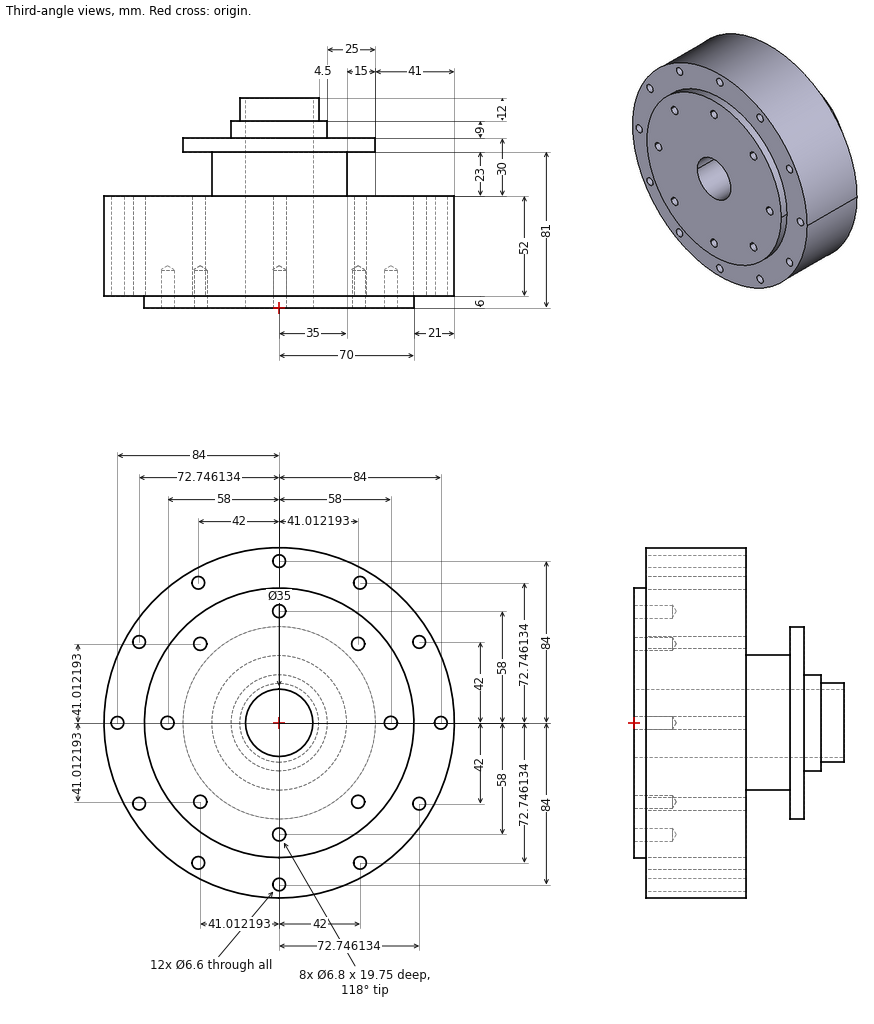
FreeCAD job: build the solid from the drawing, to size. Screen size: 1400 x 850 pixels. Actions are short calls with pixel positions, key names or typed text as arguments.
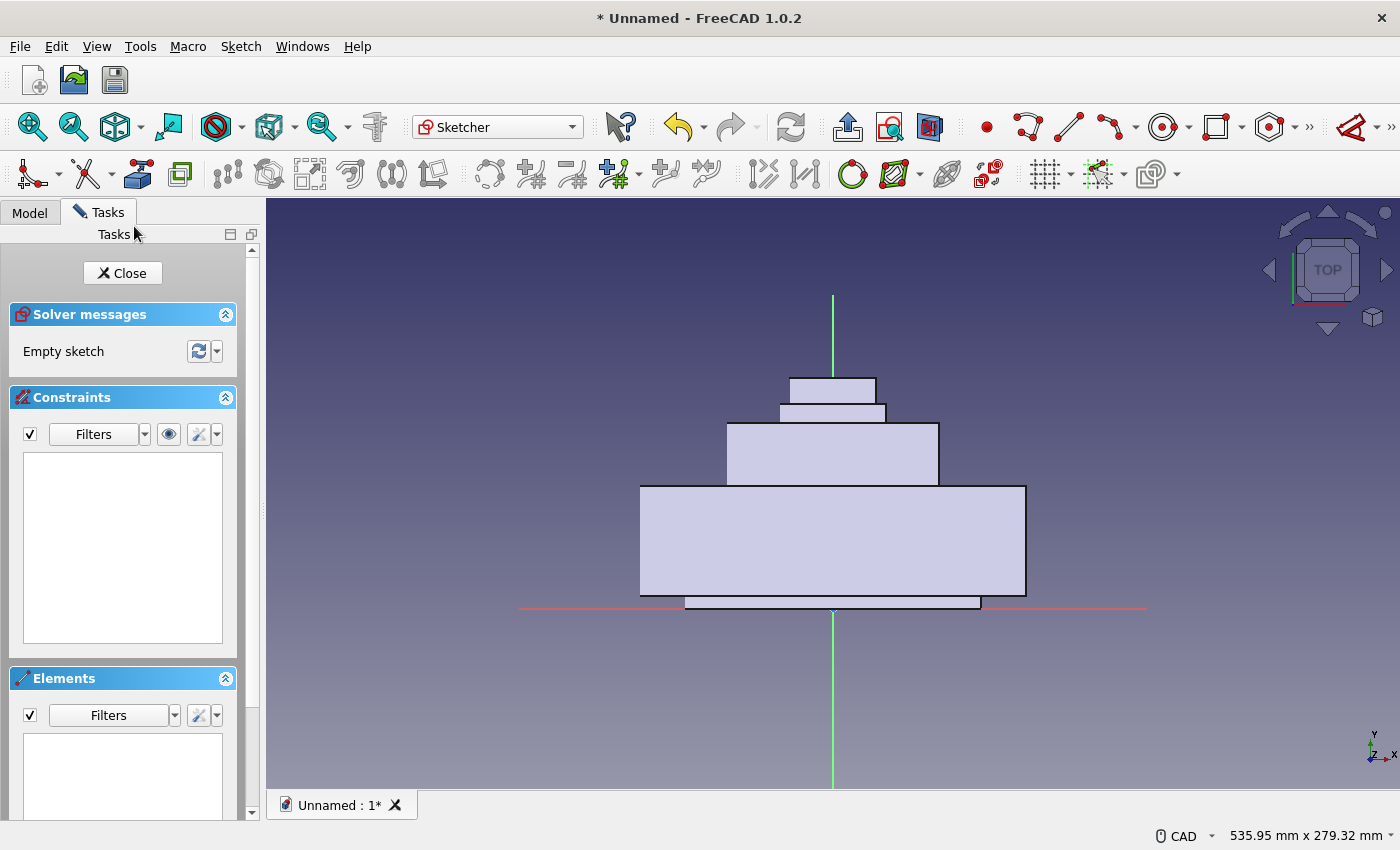
key(q)
key(s)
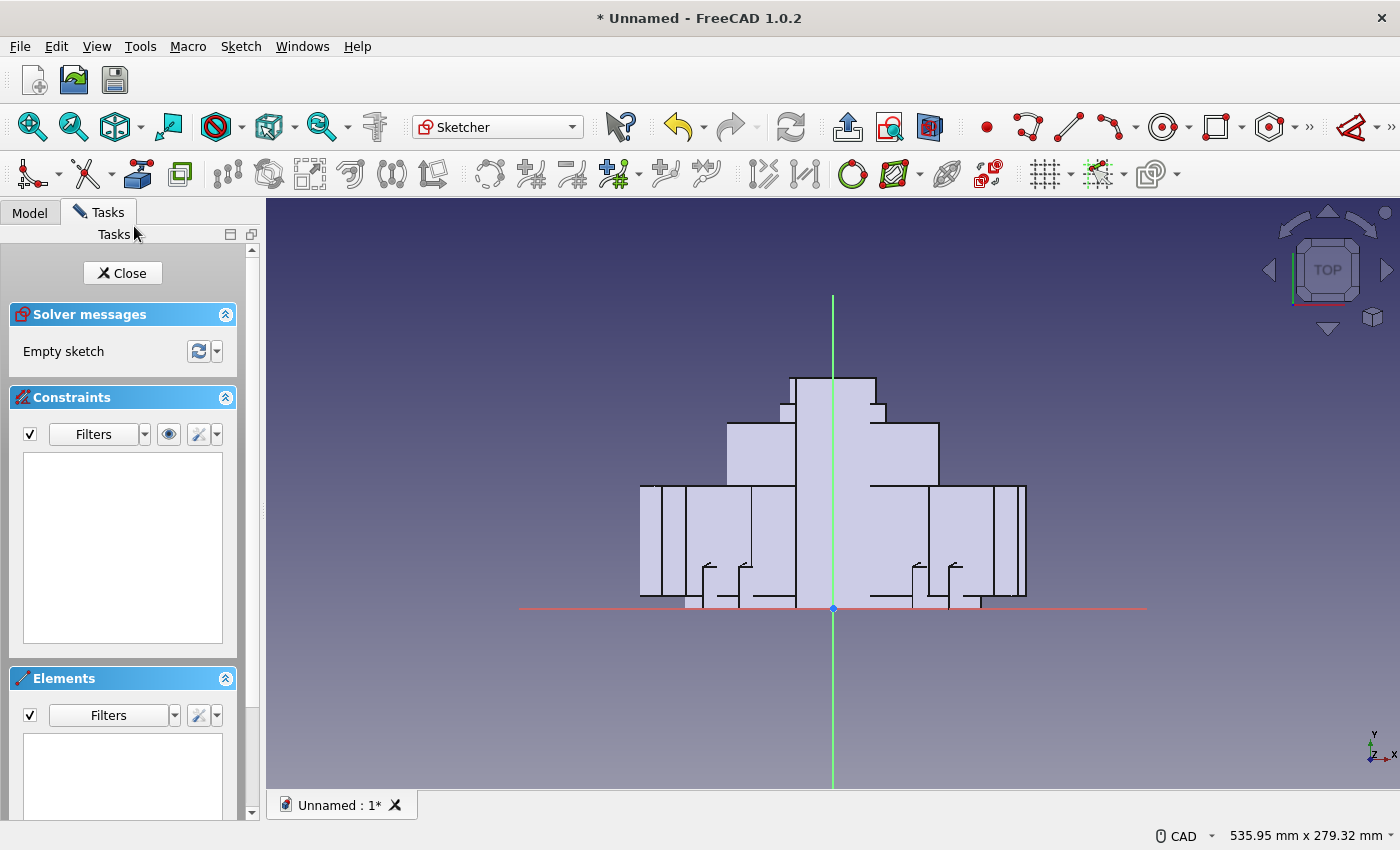
scroll(948, 457, up, 10)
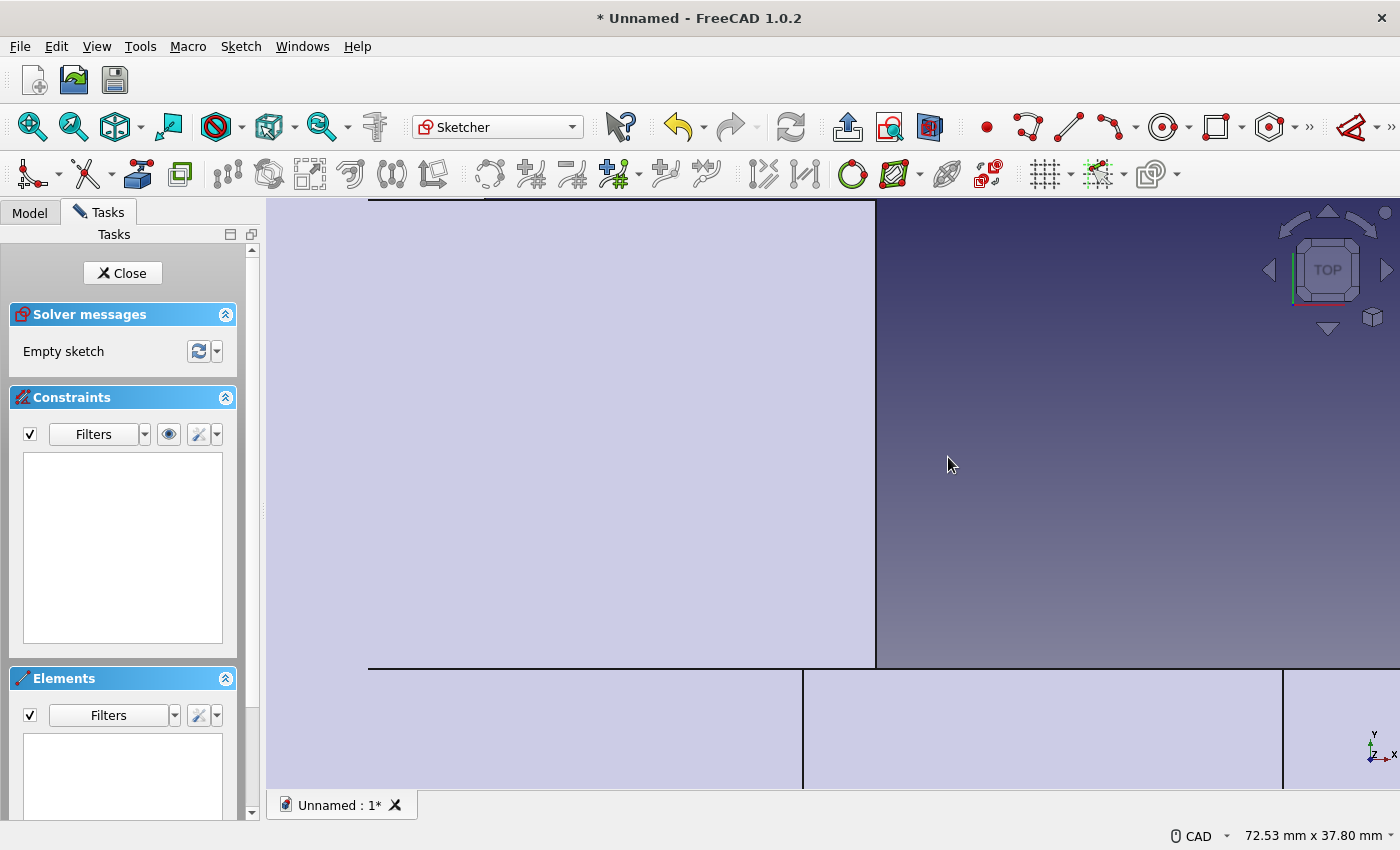
click(1216, 128)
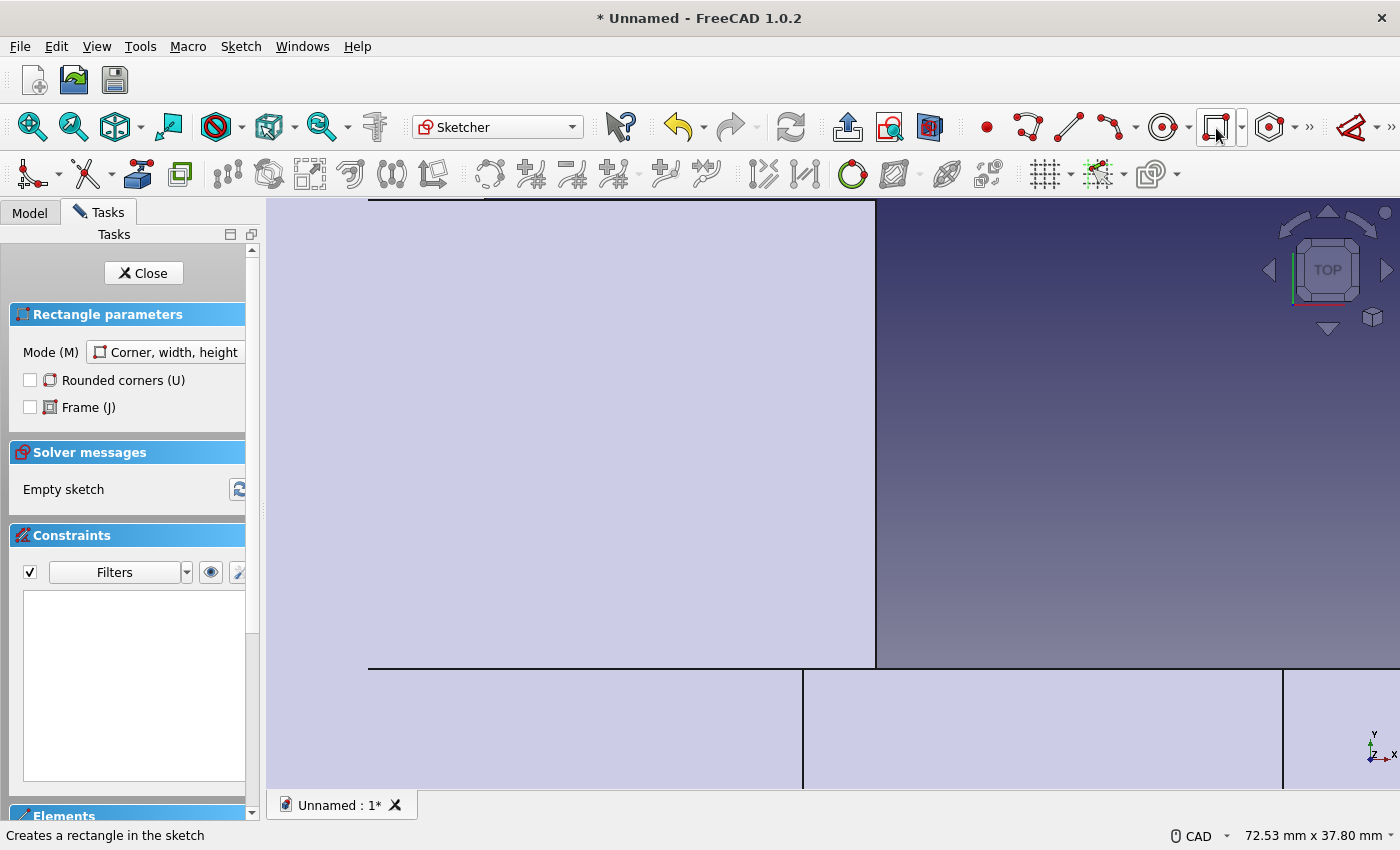
click(642, 310)
click(876, 669)
key(Escape)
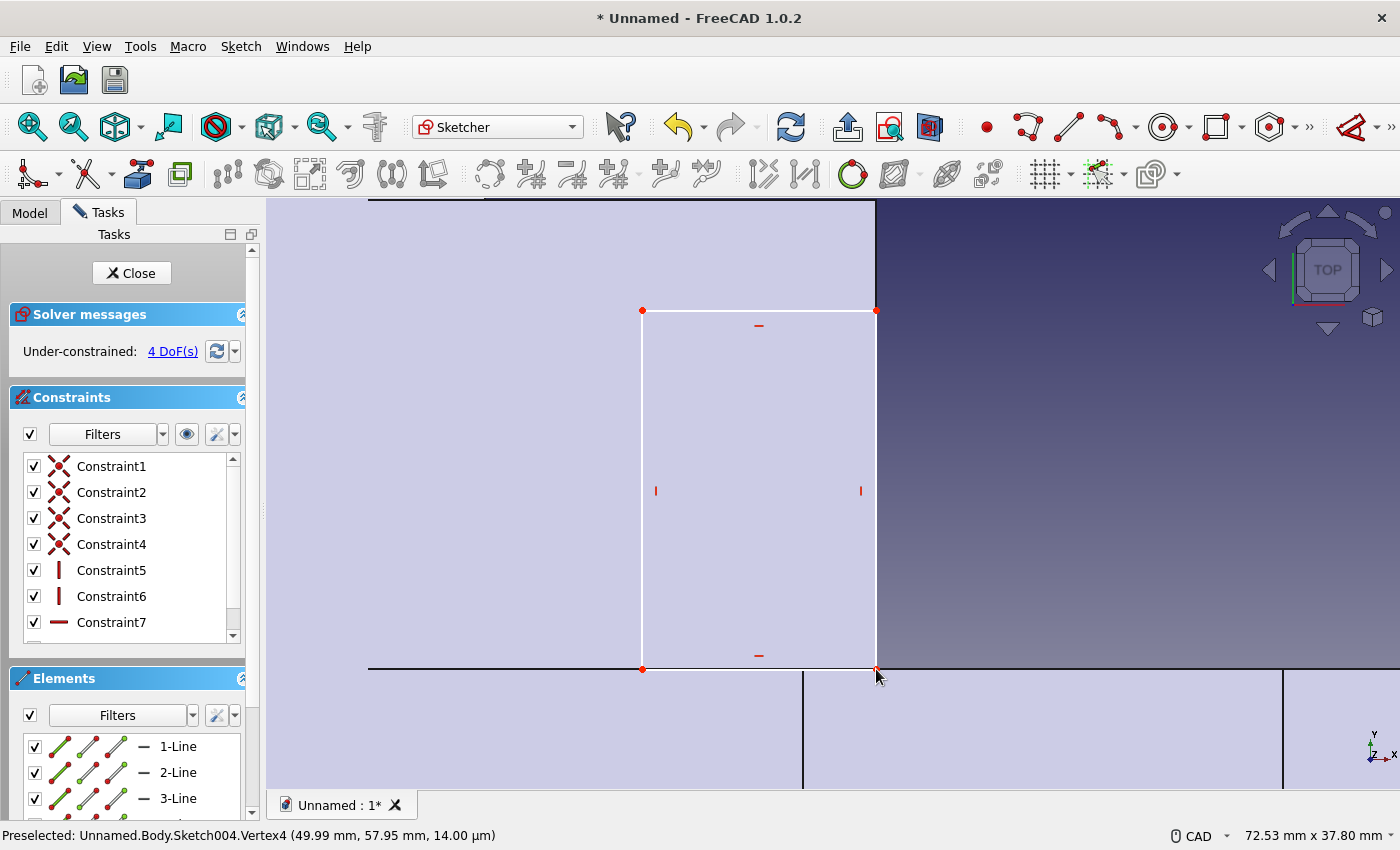
key(d)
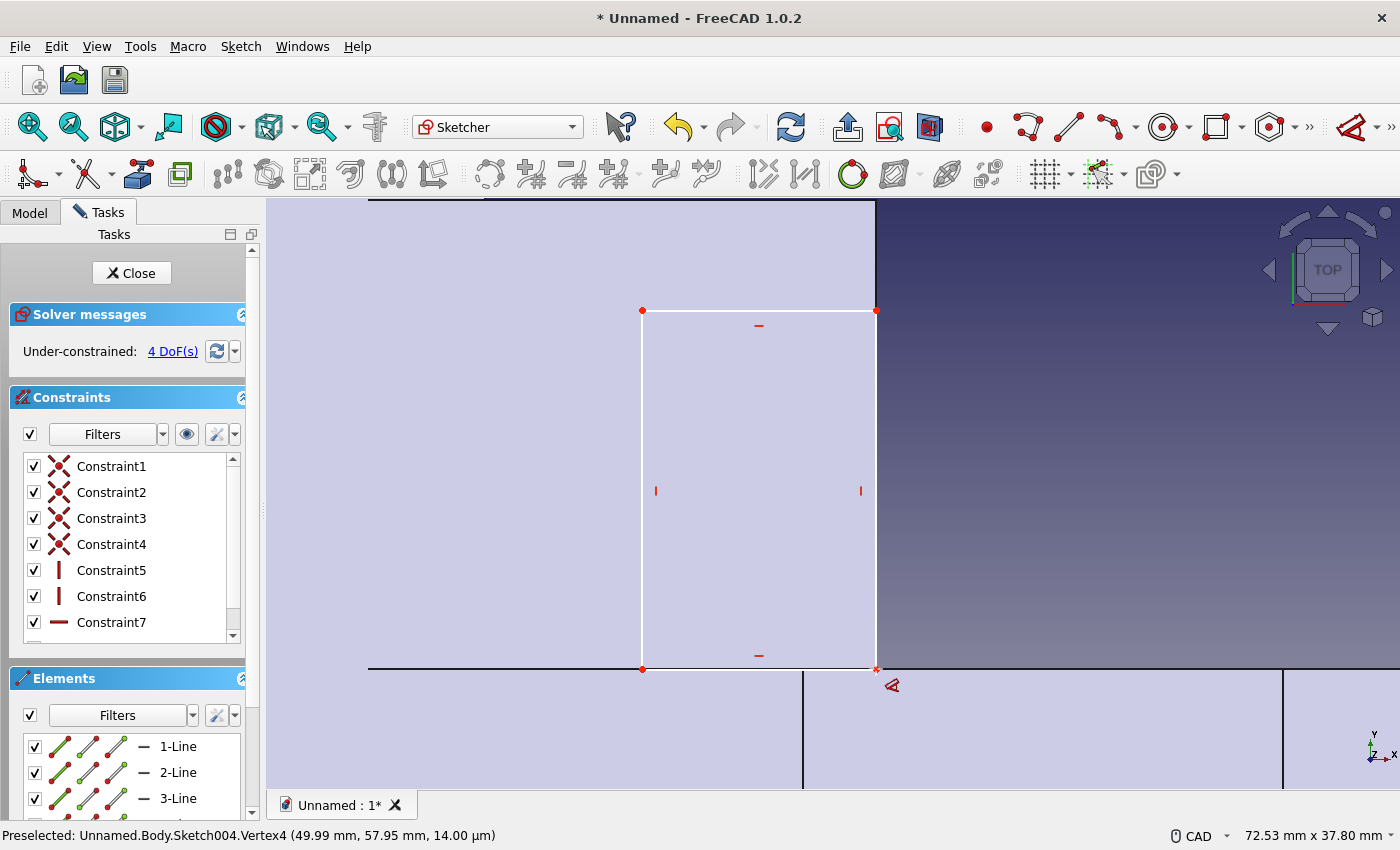
click(642, 419)
click(608, 490)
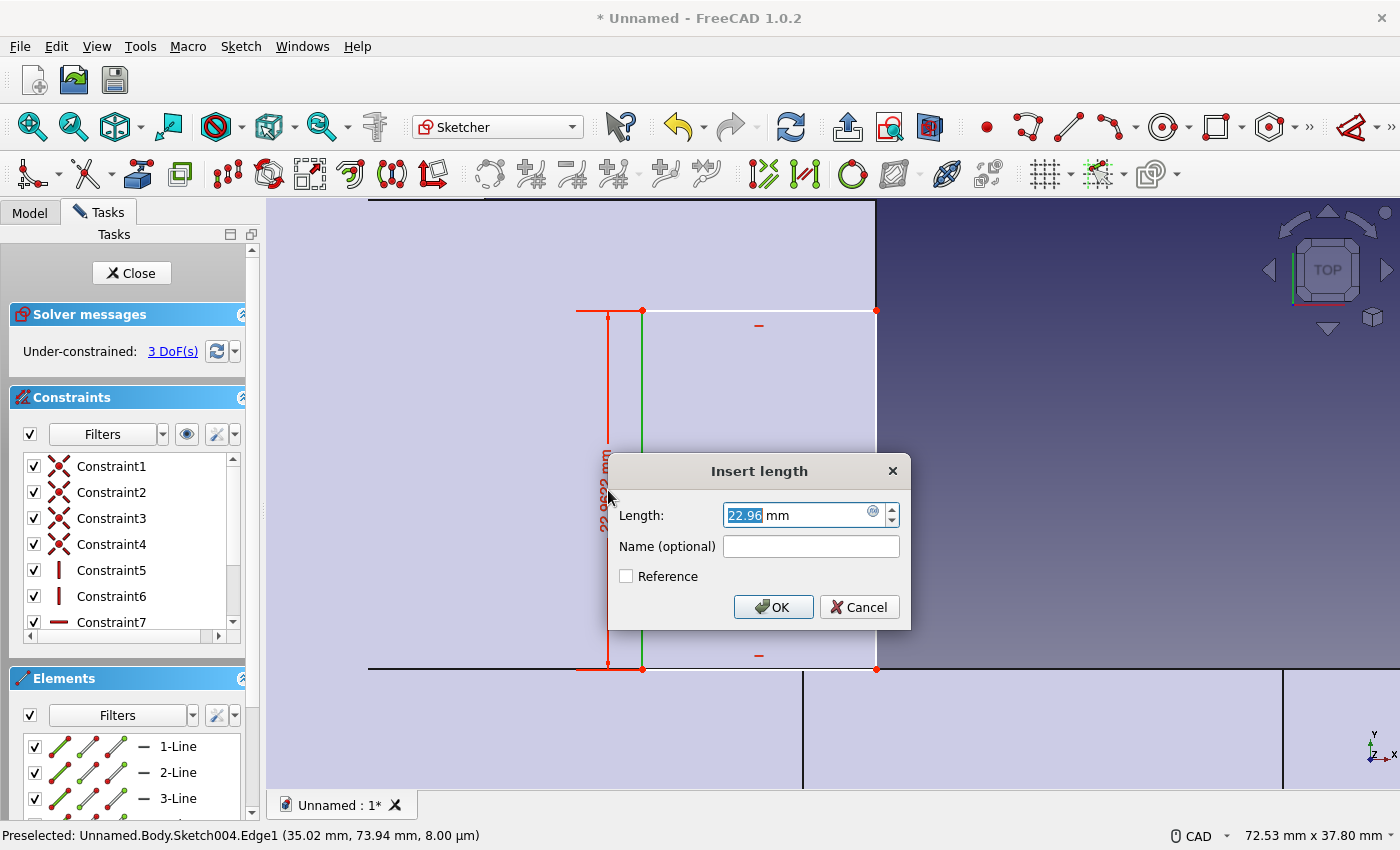
text(23)
key(Return)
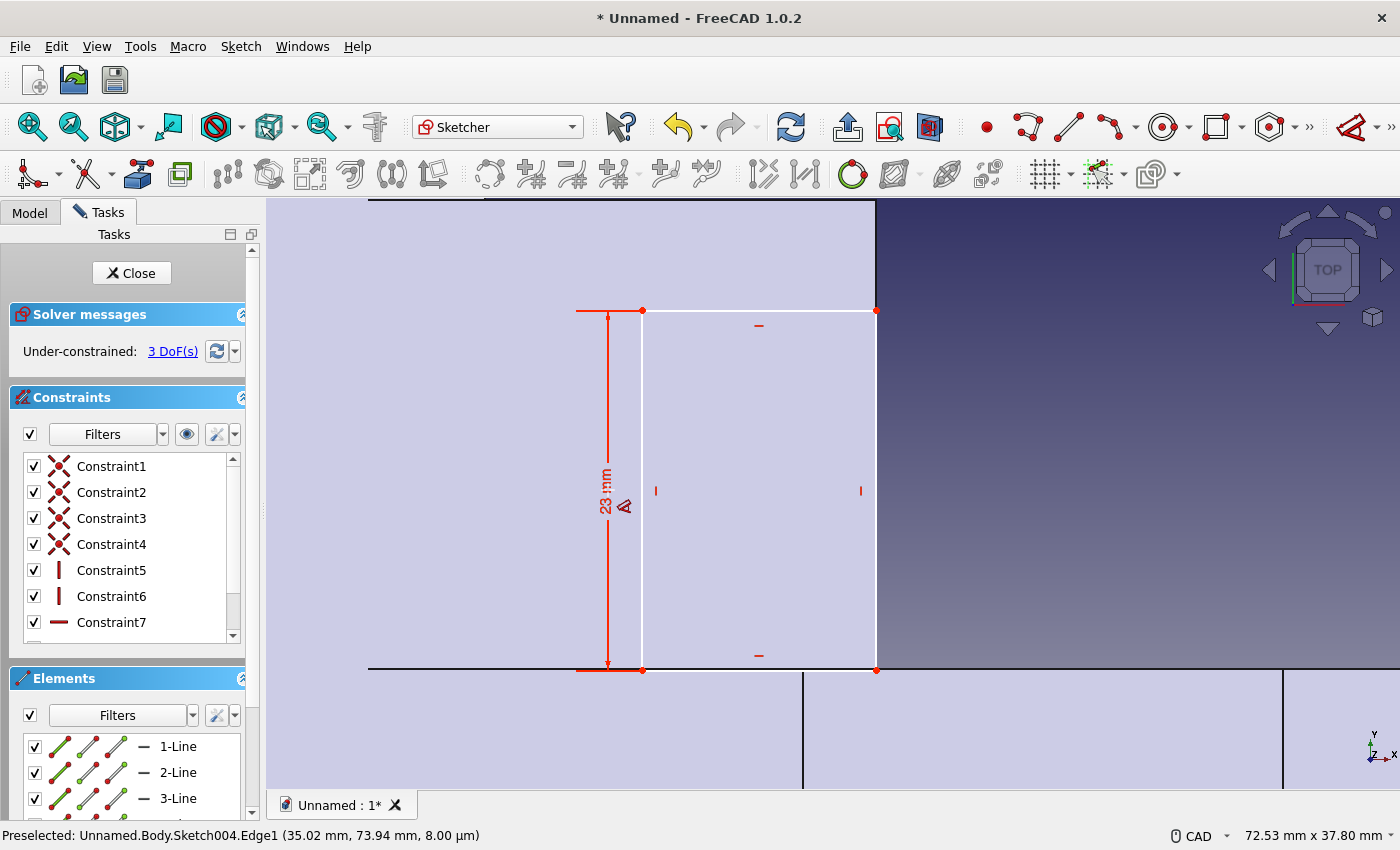
click(712, 671)
click(759, 705)